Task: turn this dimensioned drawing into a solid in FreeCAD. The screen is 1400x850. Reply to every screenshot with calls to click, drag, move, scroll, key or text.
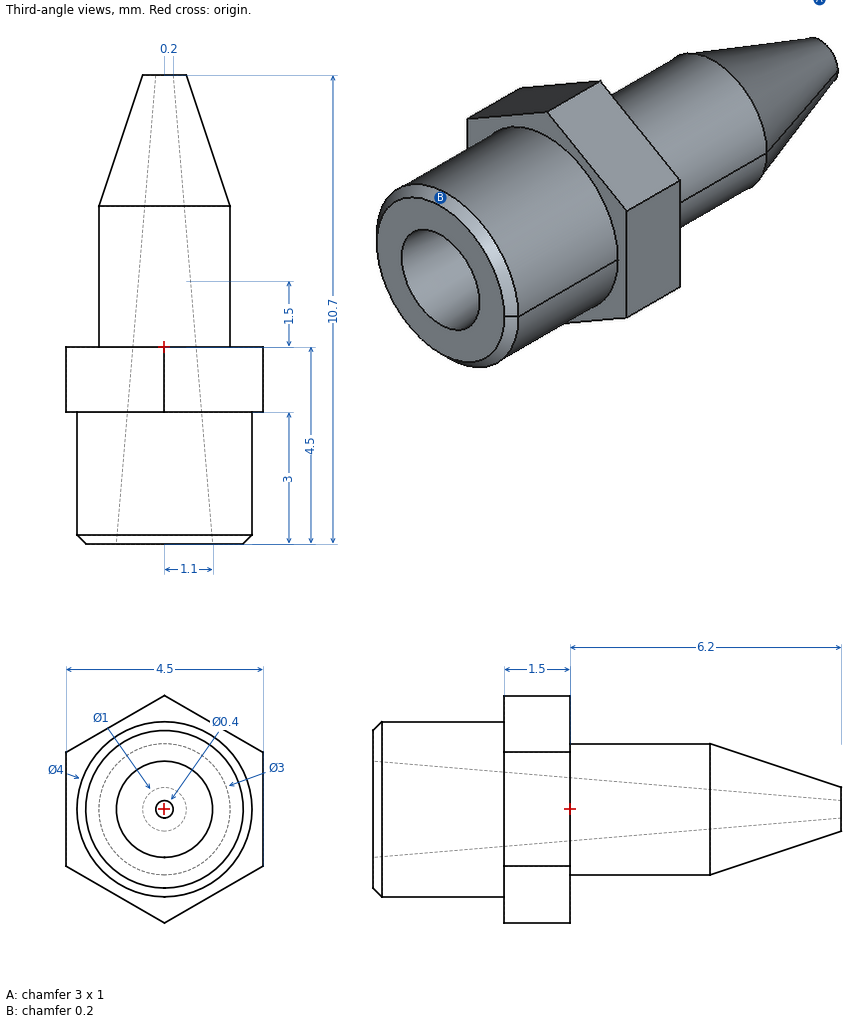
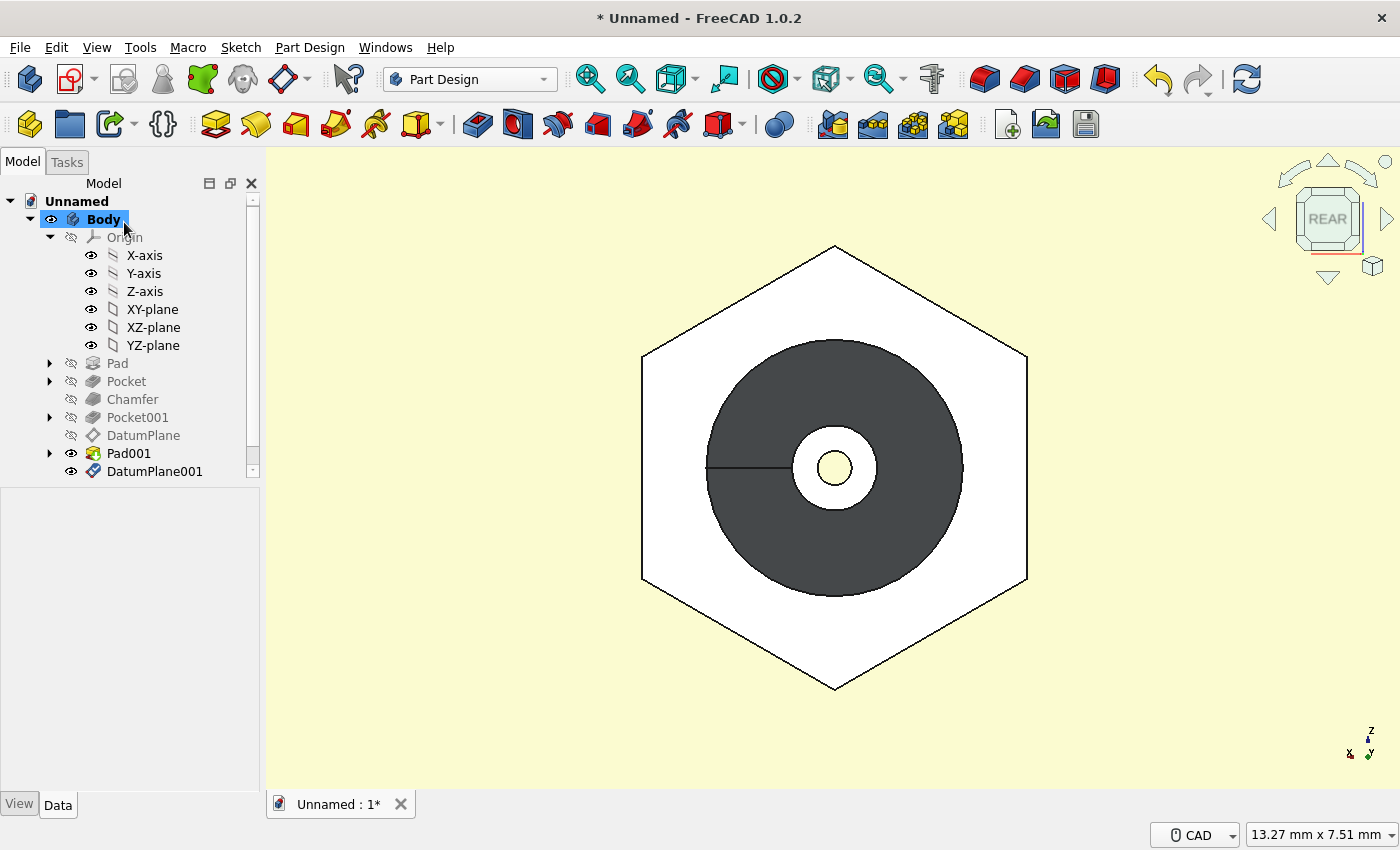
click(116, 471)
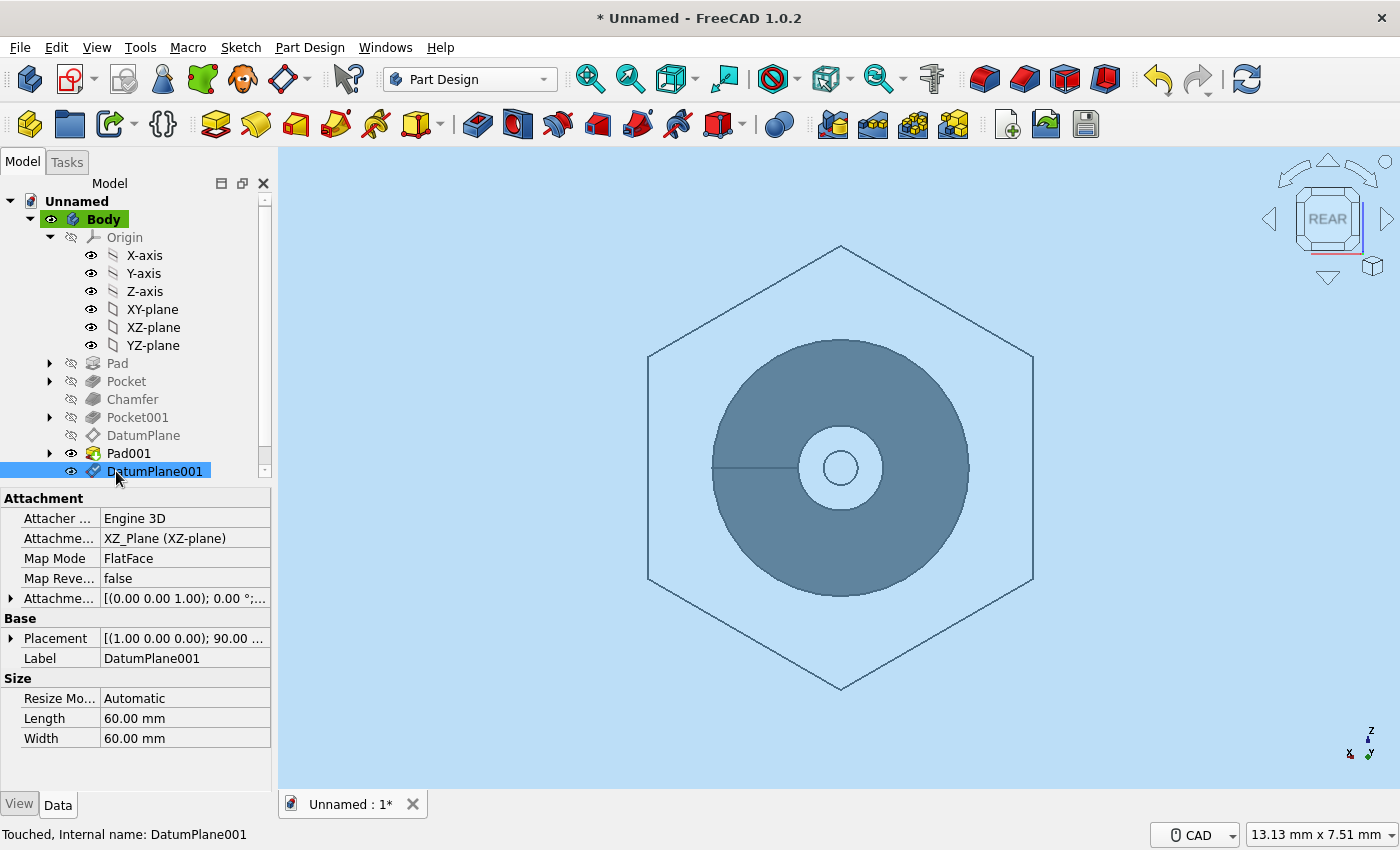
click(70, 80)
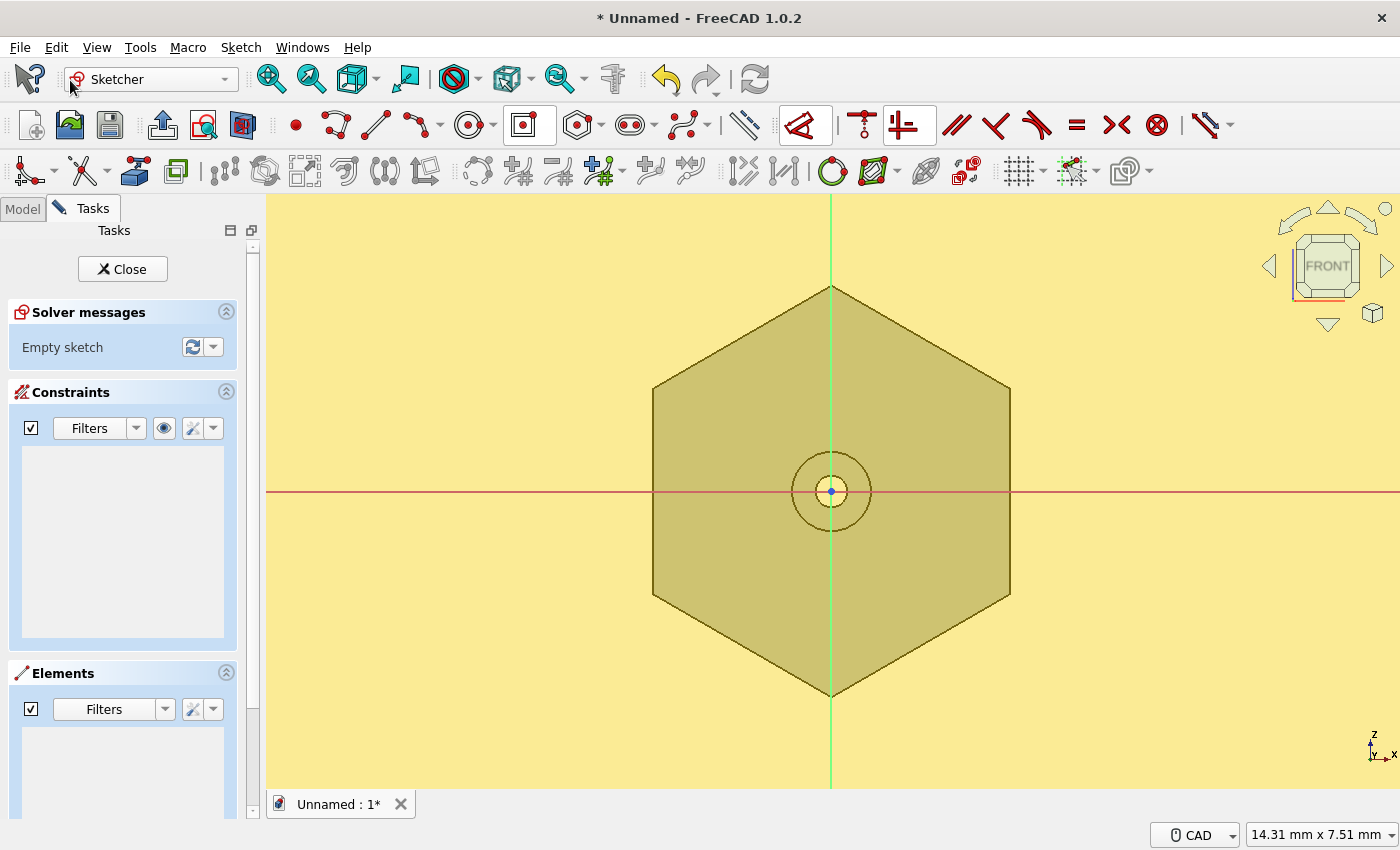
click(470, 126)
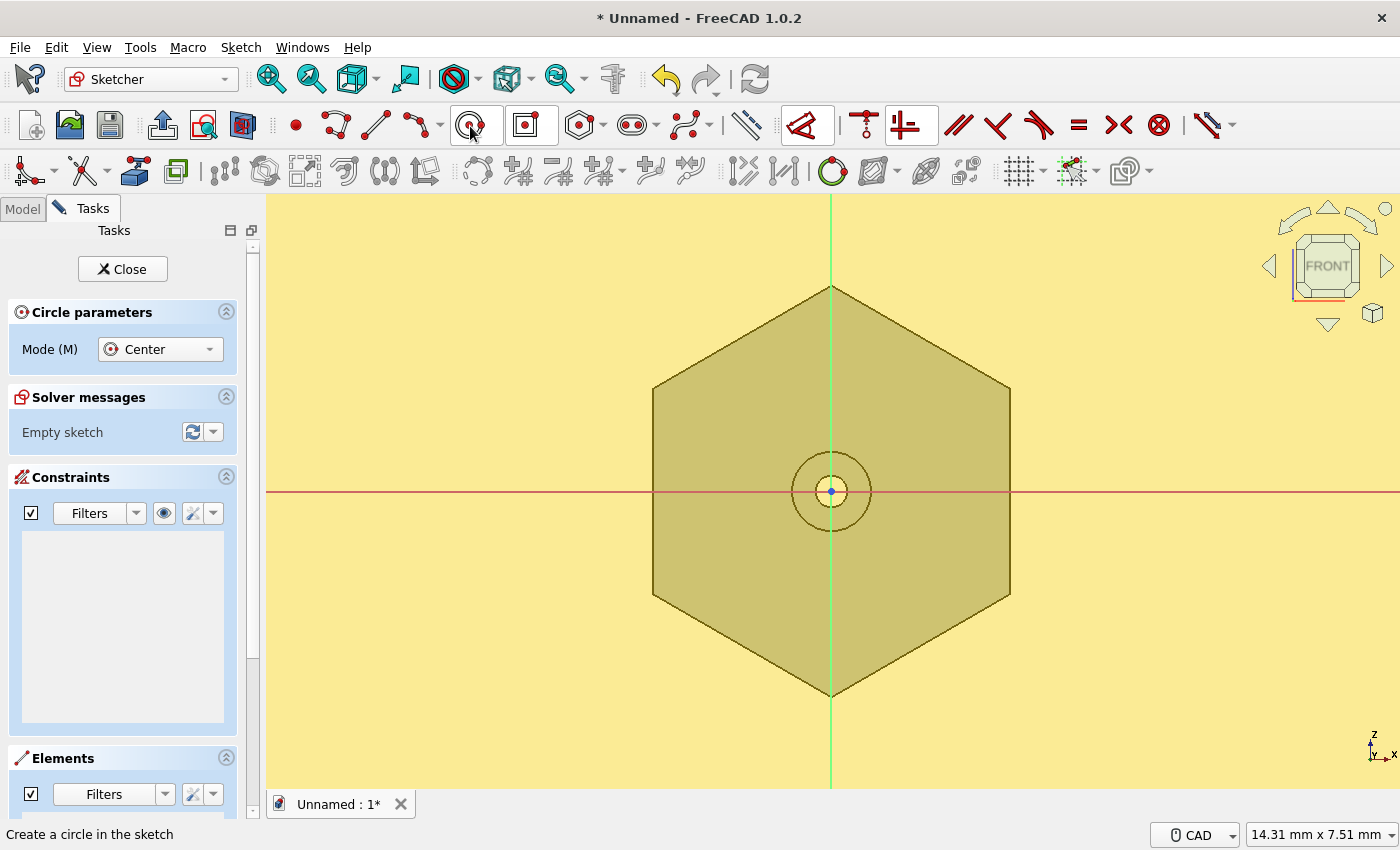
click(832, 492)
click(944, 379)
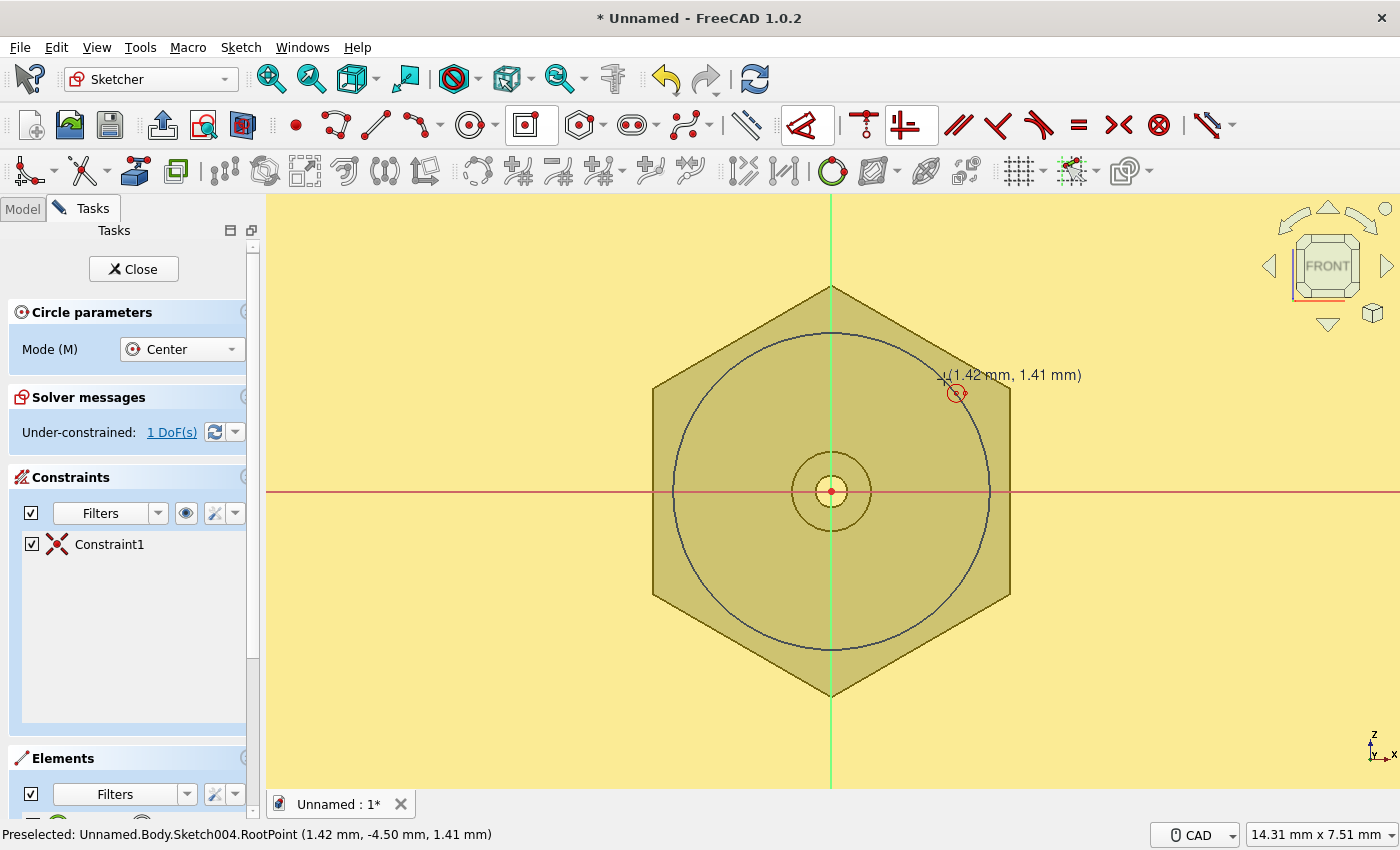
click(832, 492)
click(860, 463)
key(Escape)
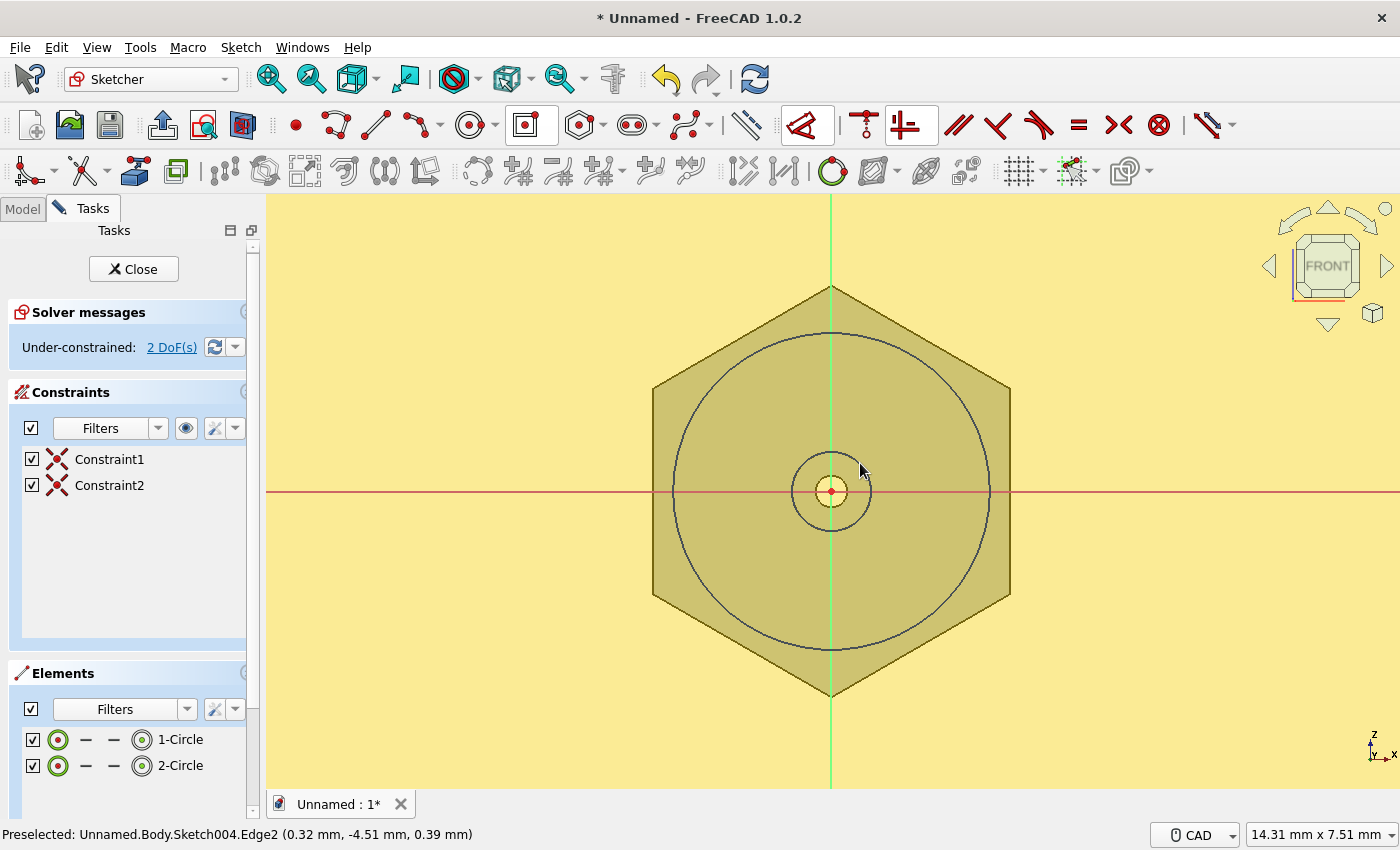
click(943, 379)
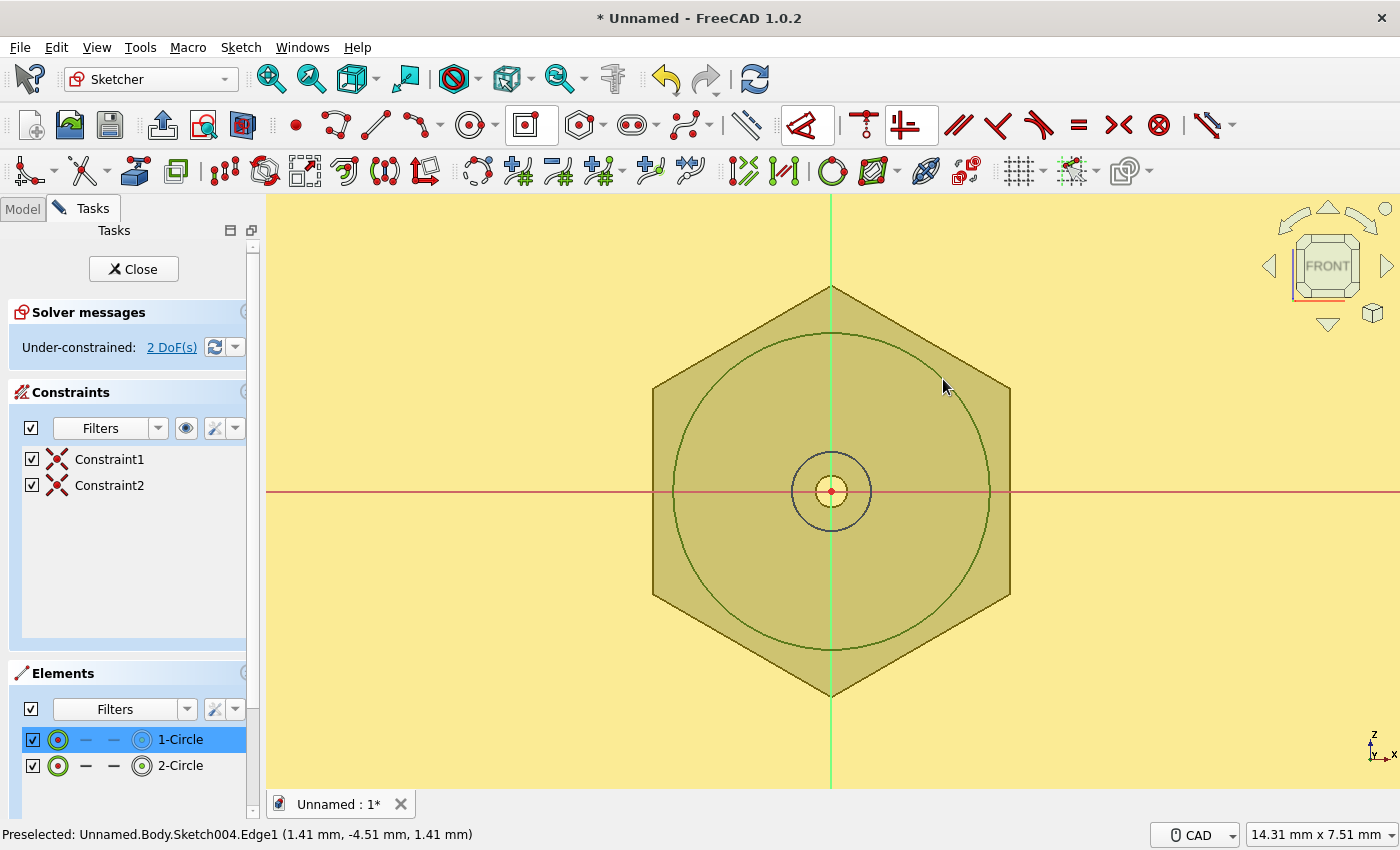
key(k)
key(o)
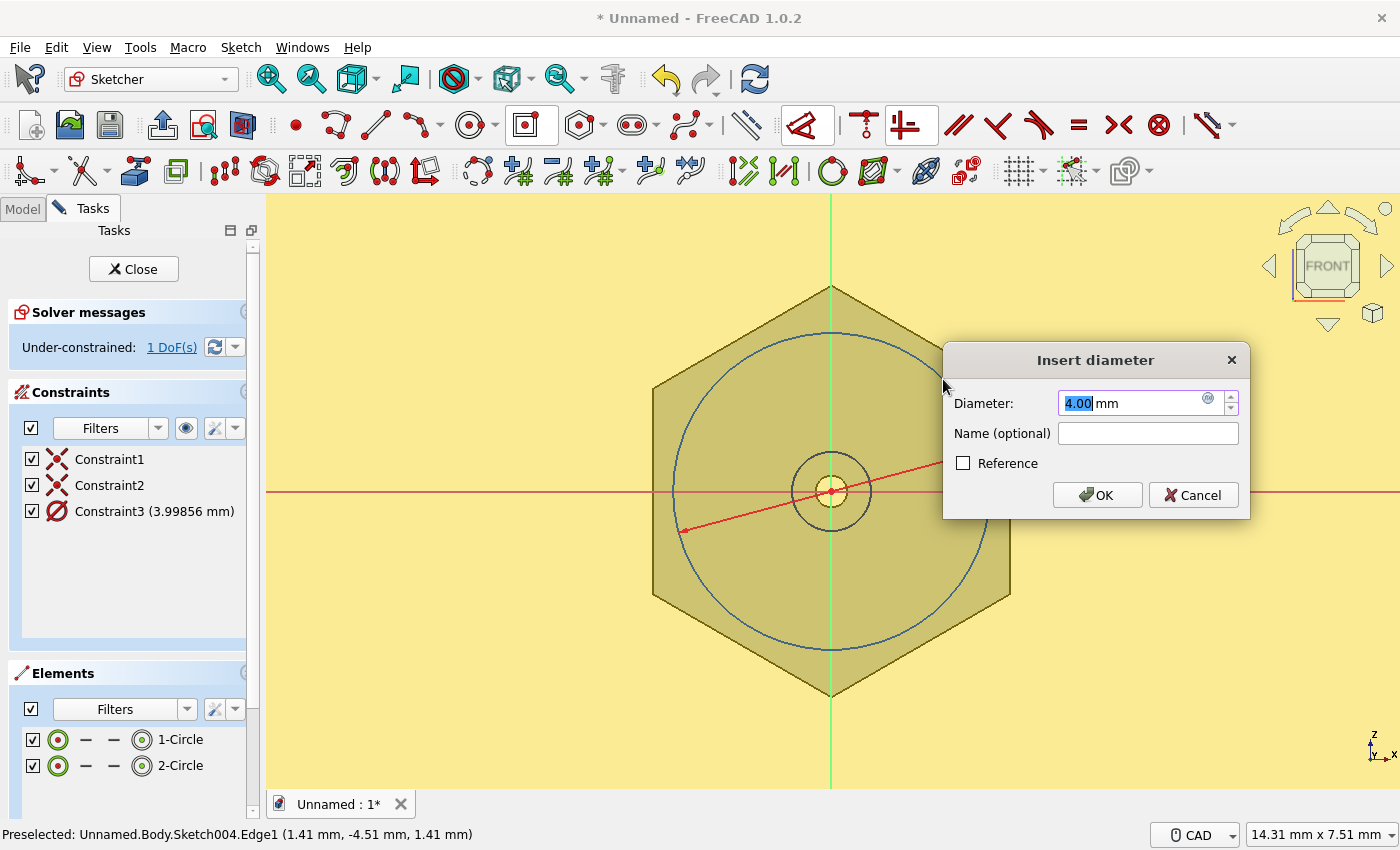
text(4)
key(Return)